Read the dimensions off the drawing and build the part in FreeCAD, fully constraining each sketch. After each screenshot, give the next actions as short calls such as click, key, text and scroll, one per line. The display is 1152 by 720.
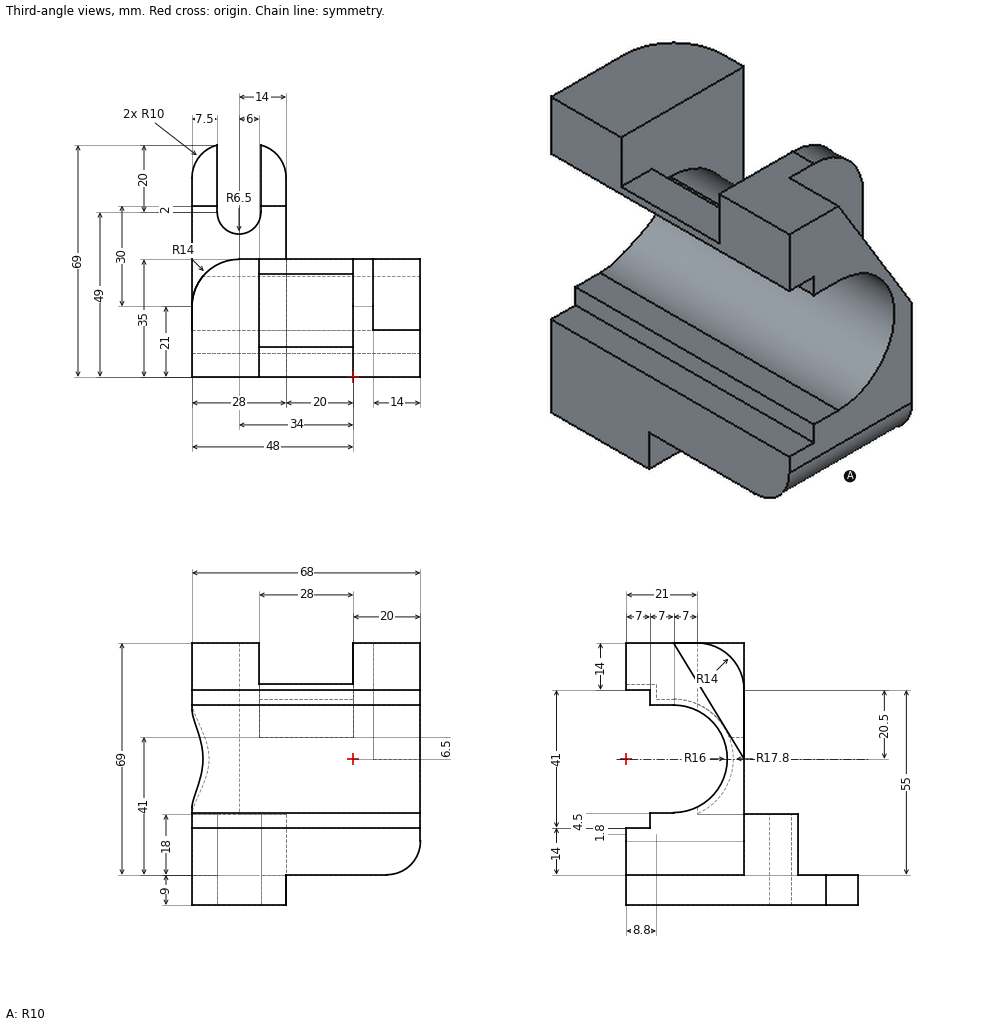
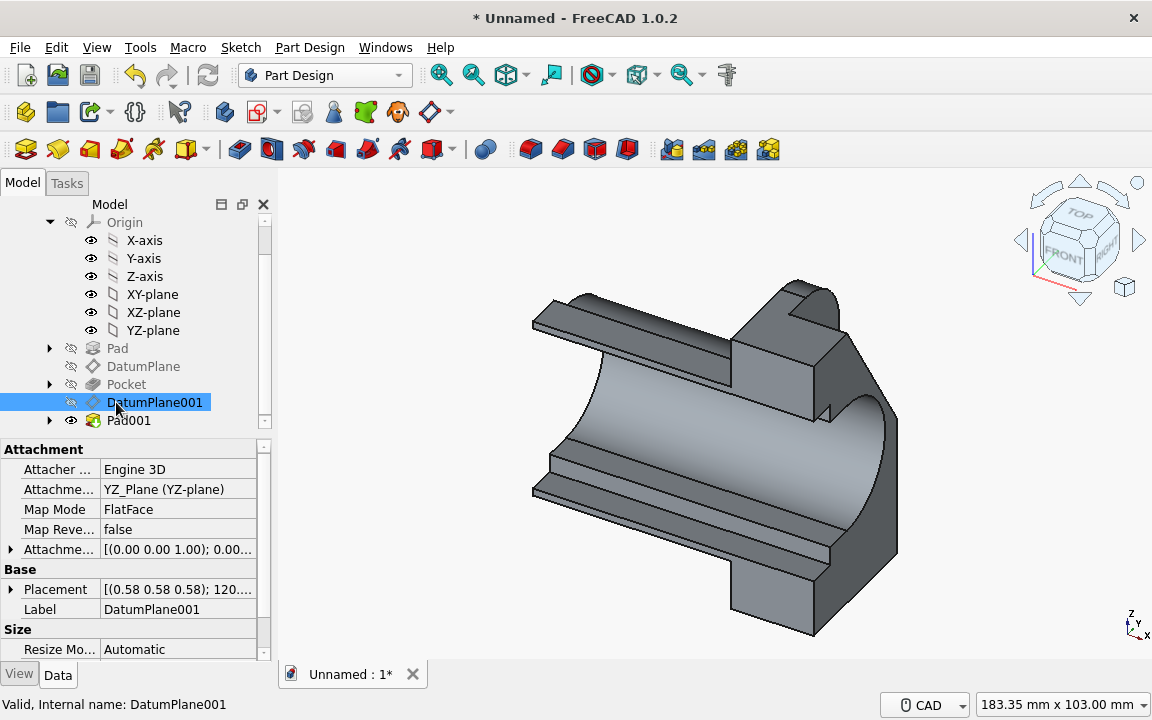
click(778, 330)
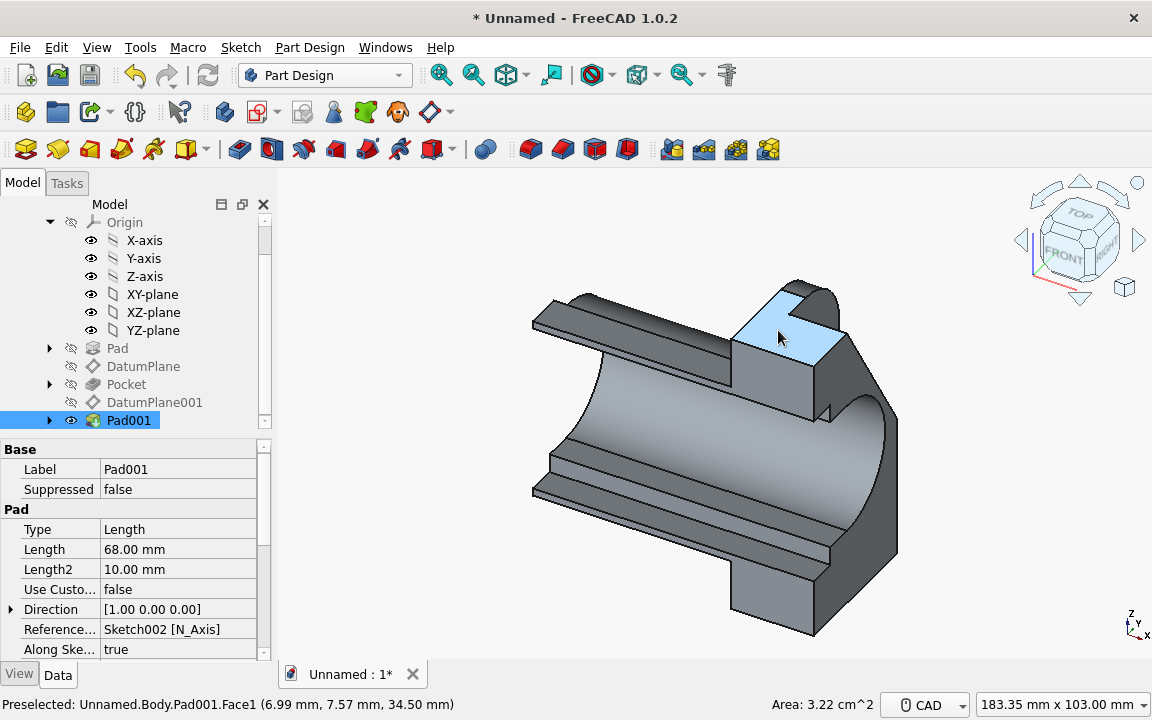
click(258, 112)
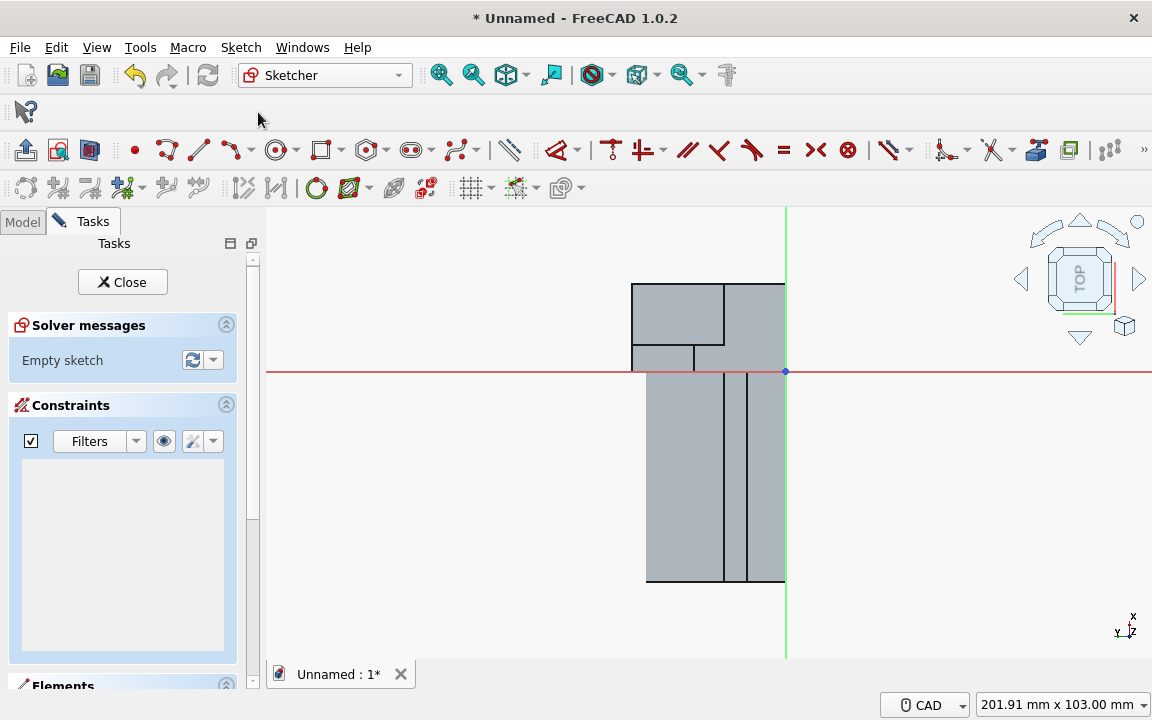
click(168, 150)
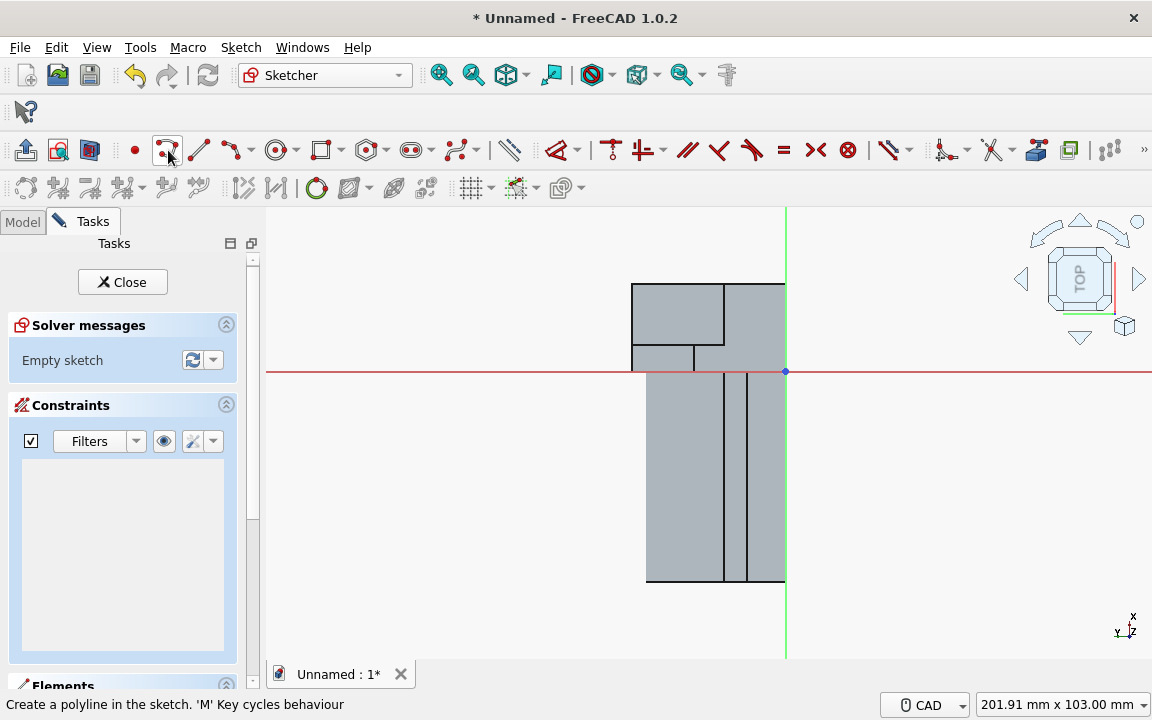
click(694, 582)
click(786, 582)
click(777, 494)
click(632, 494)
click(632, 521)
right_click(632, 521)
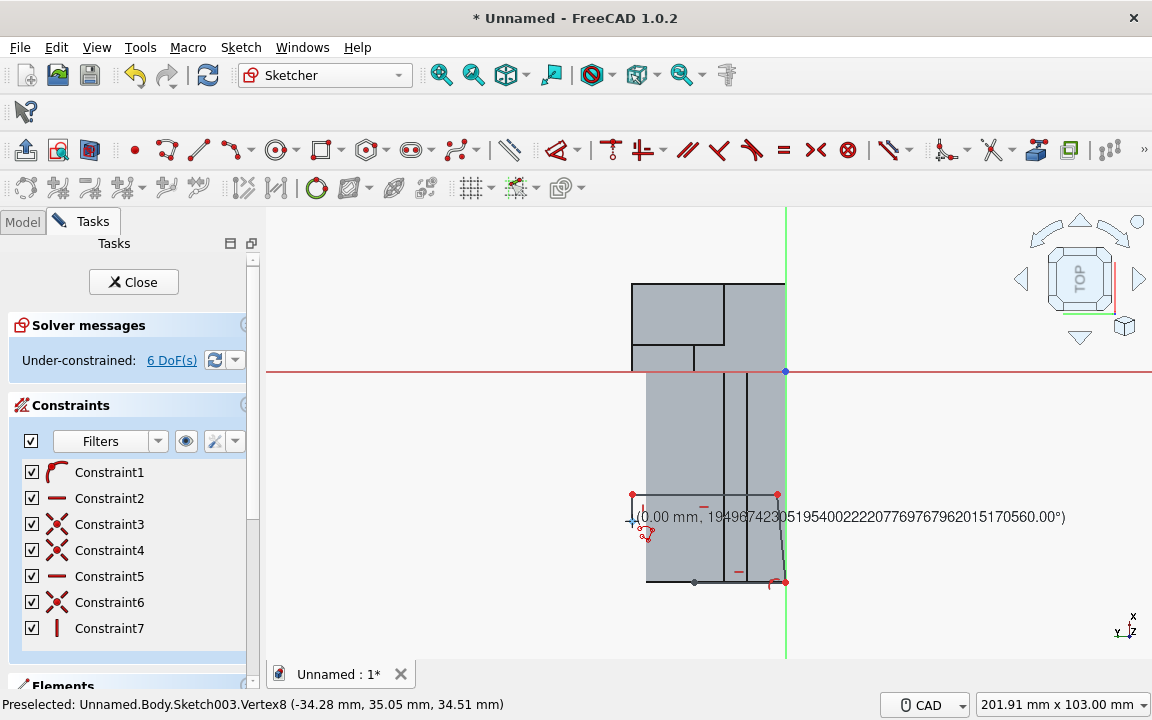
click(232, 150)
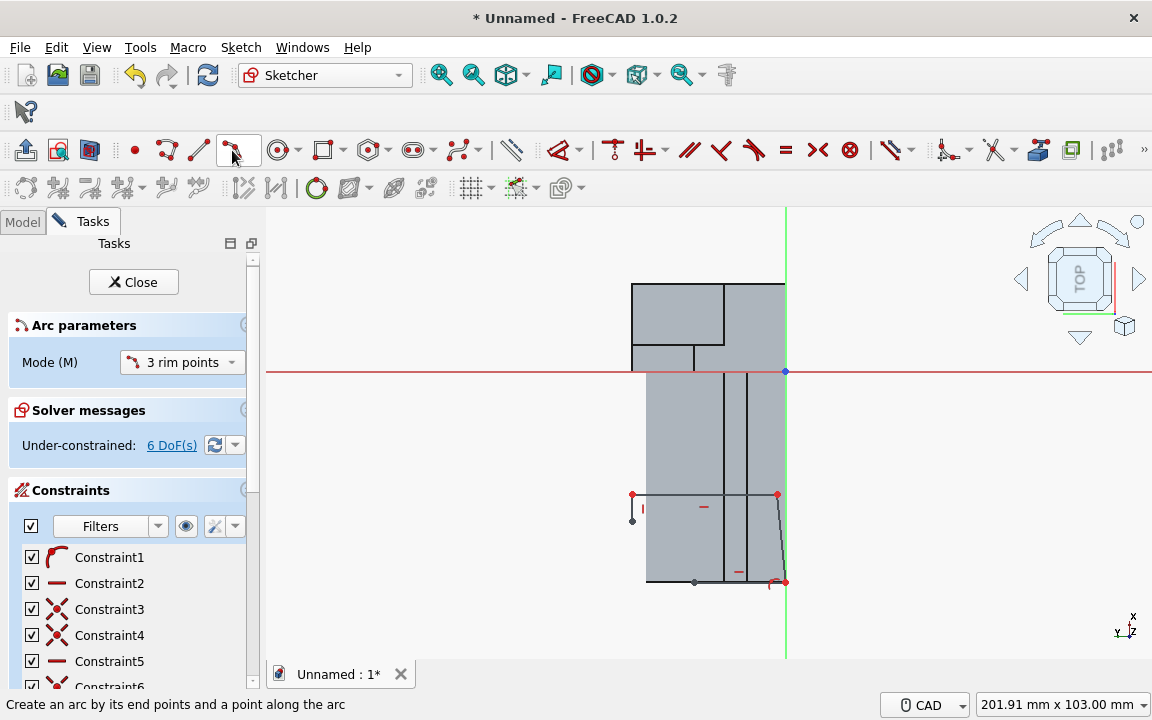
click(632, 522)
click(694, 583)
click(650, 564)
key(Escape)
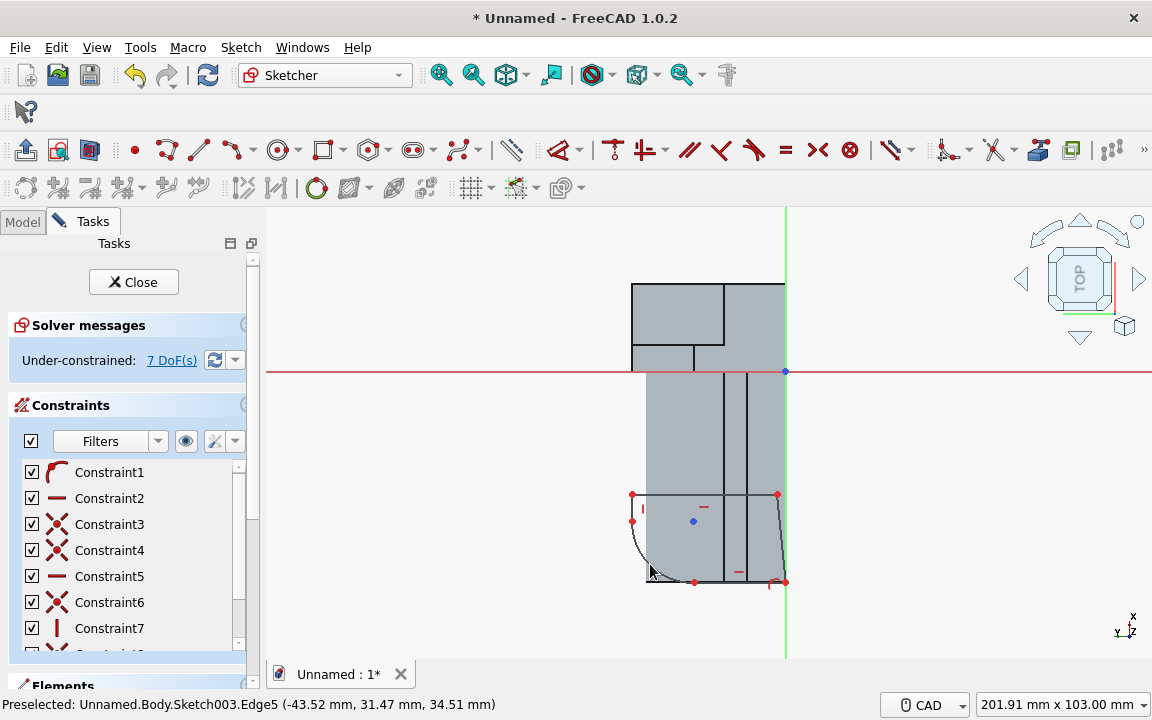
click(722, 583)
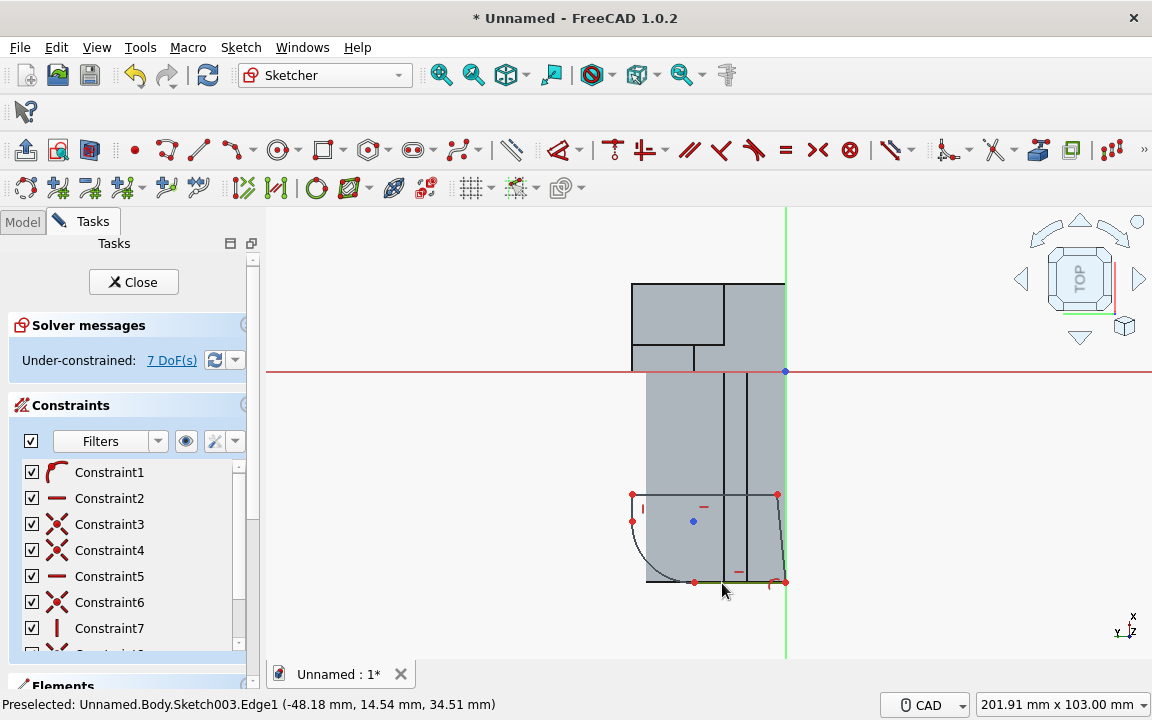
click(639, 550)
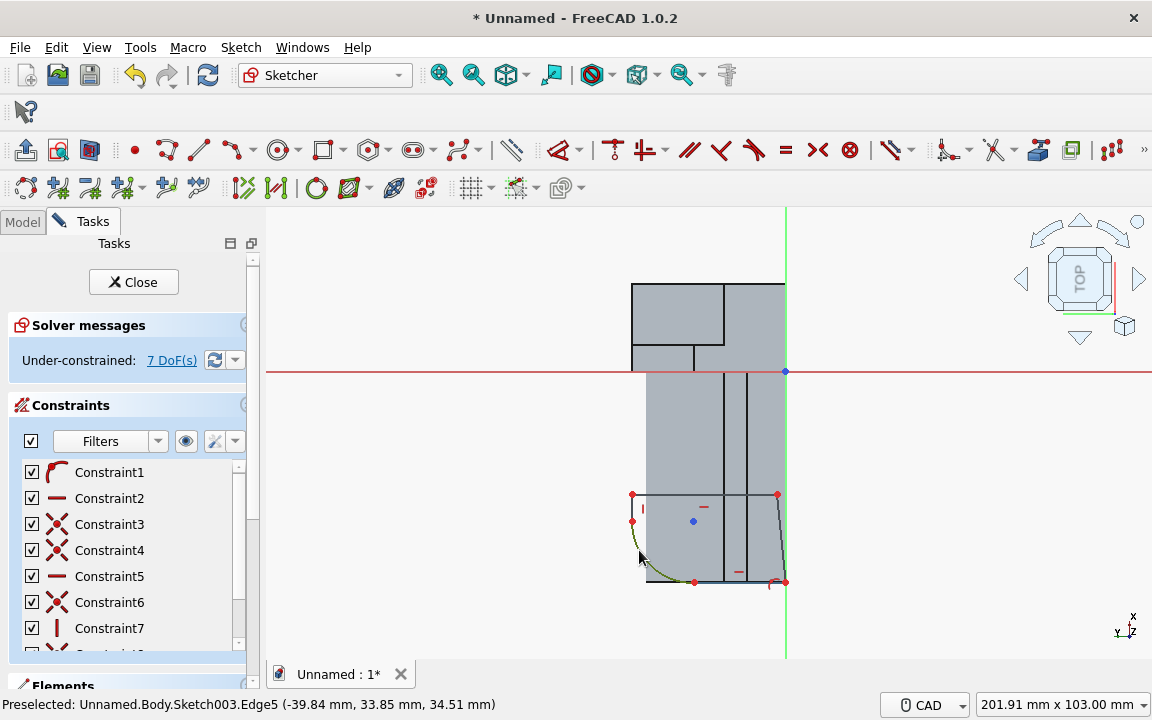
click(754, 150)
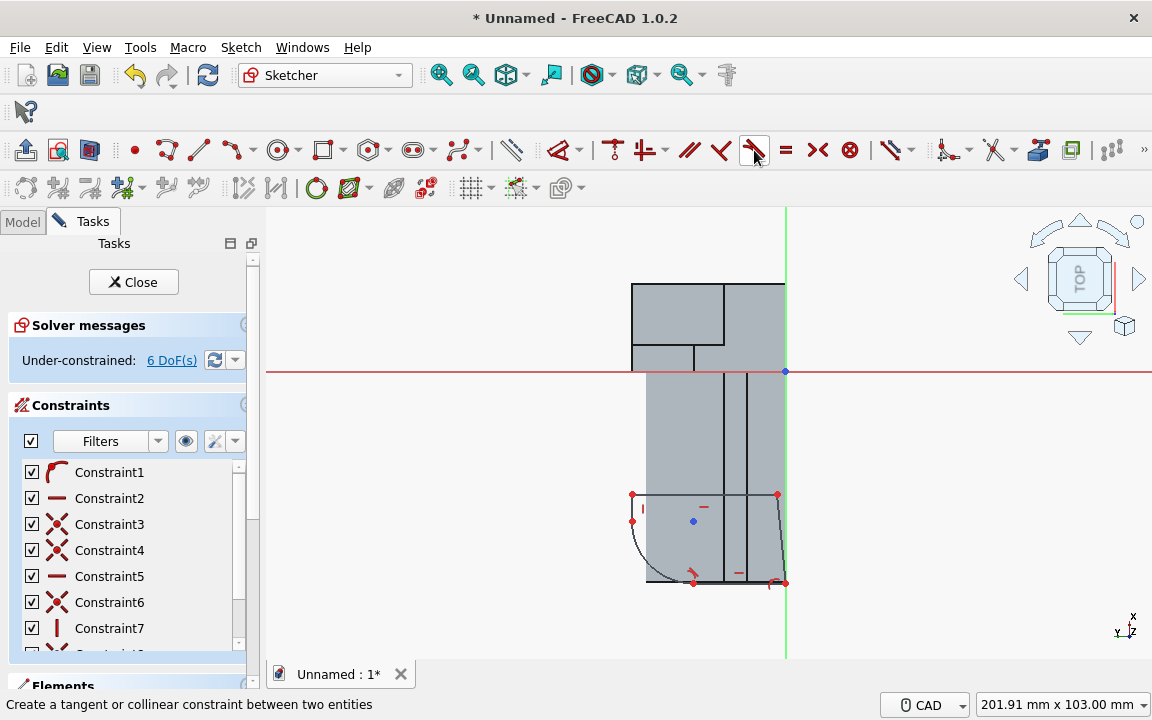
scroll(632, 506, up, 2)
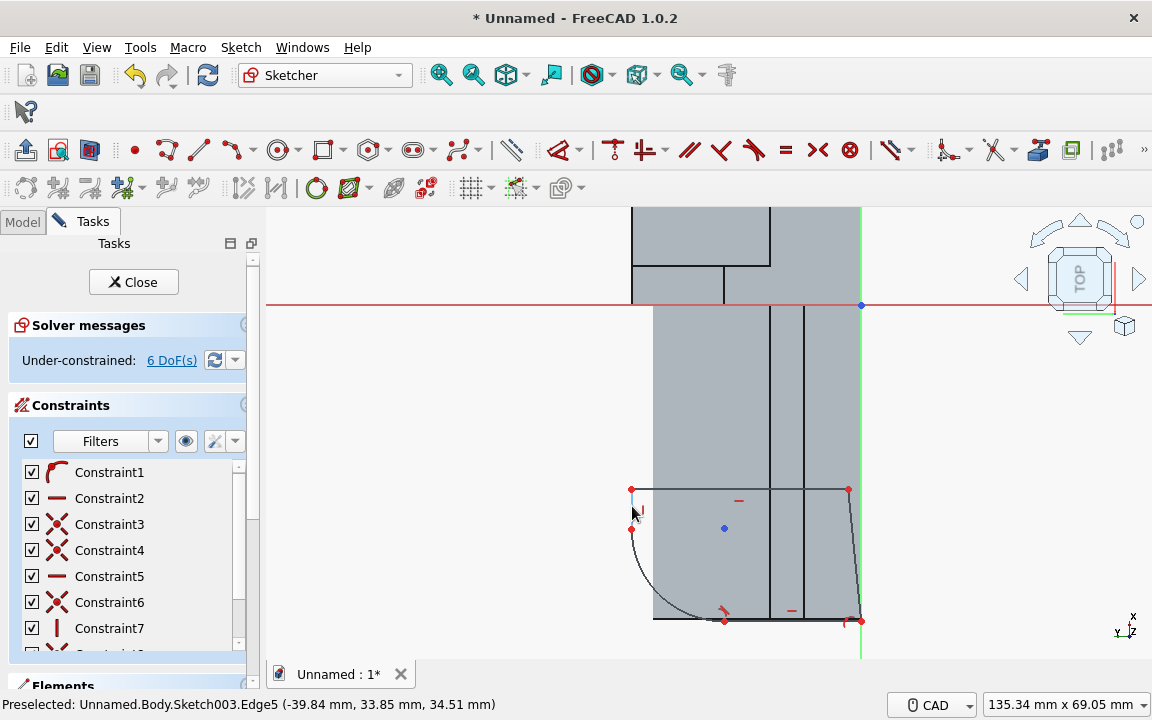
click(632, 505)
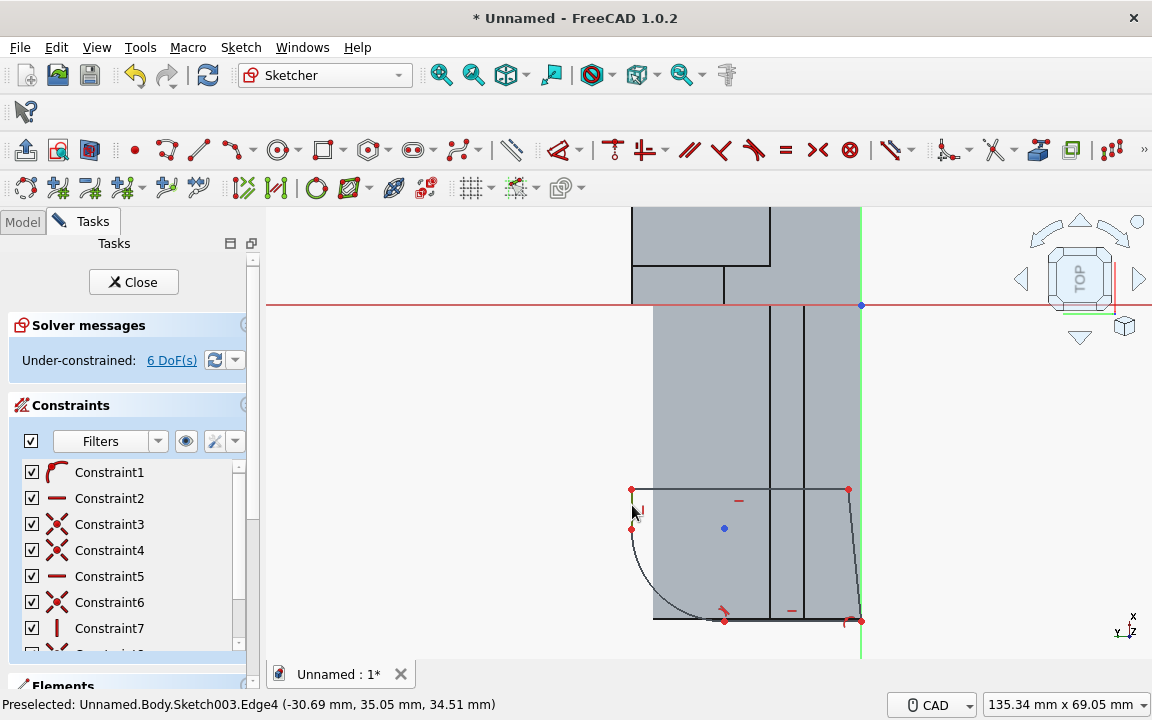
click(642, 571)